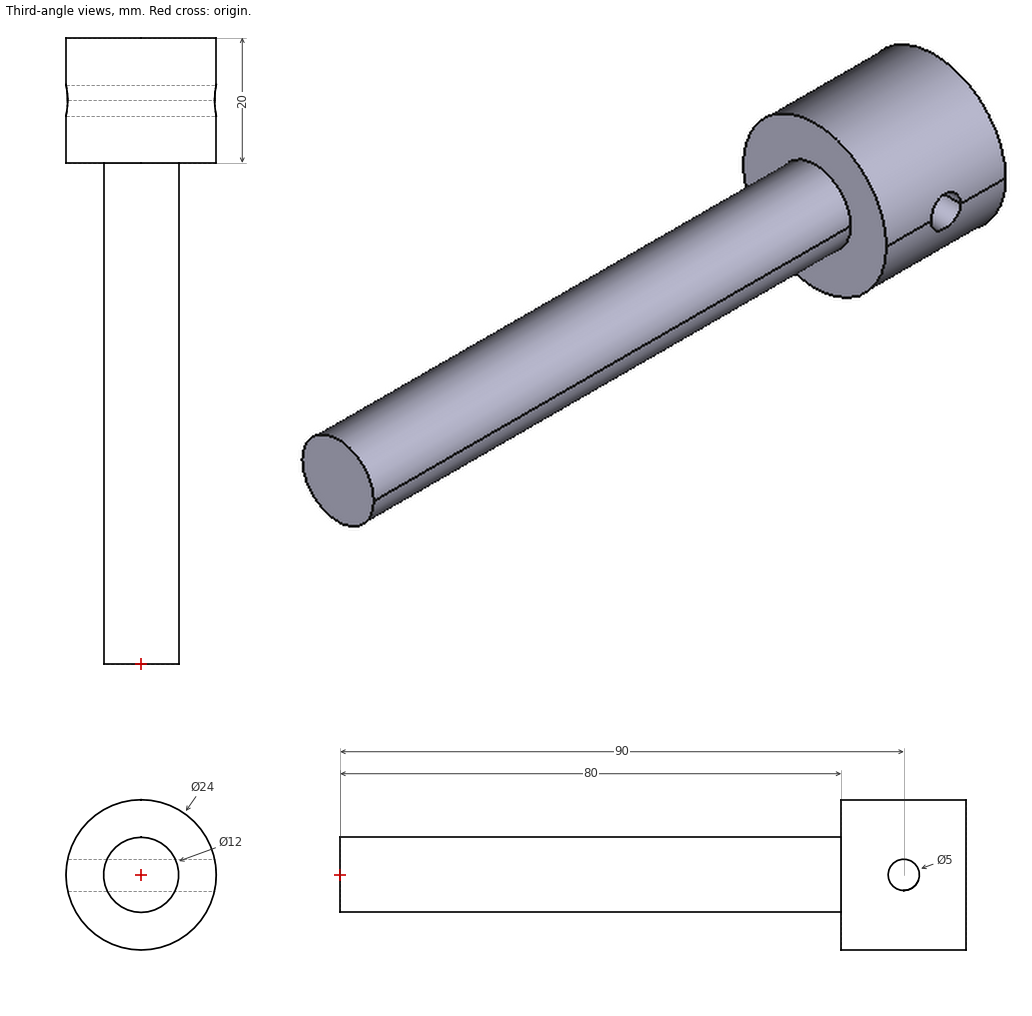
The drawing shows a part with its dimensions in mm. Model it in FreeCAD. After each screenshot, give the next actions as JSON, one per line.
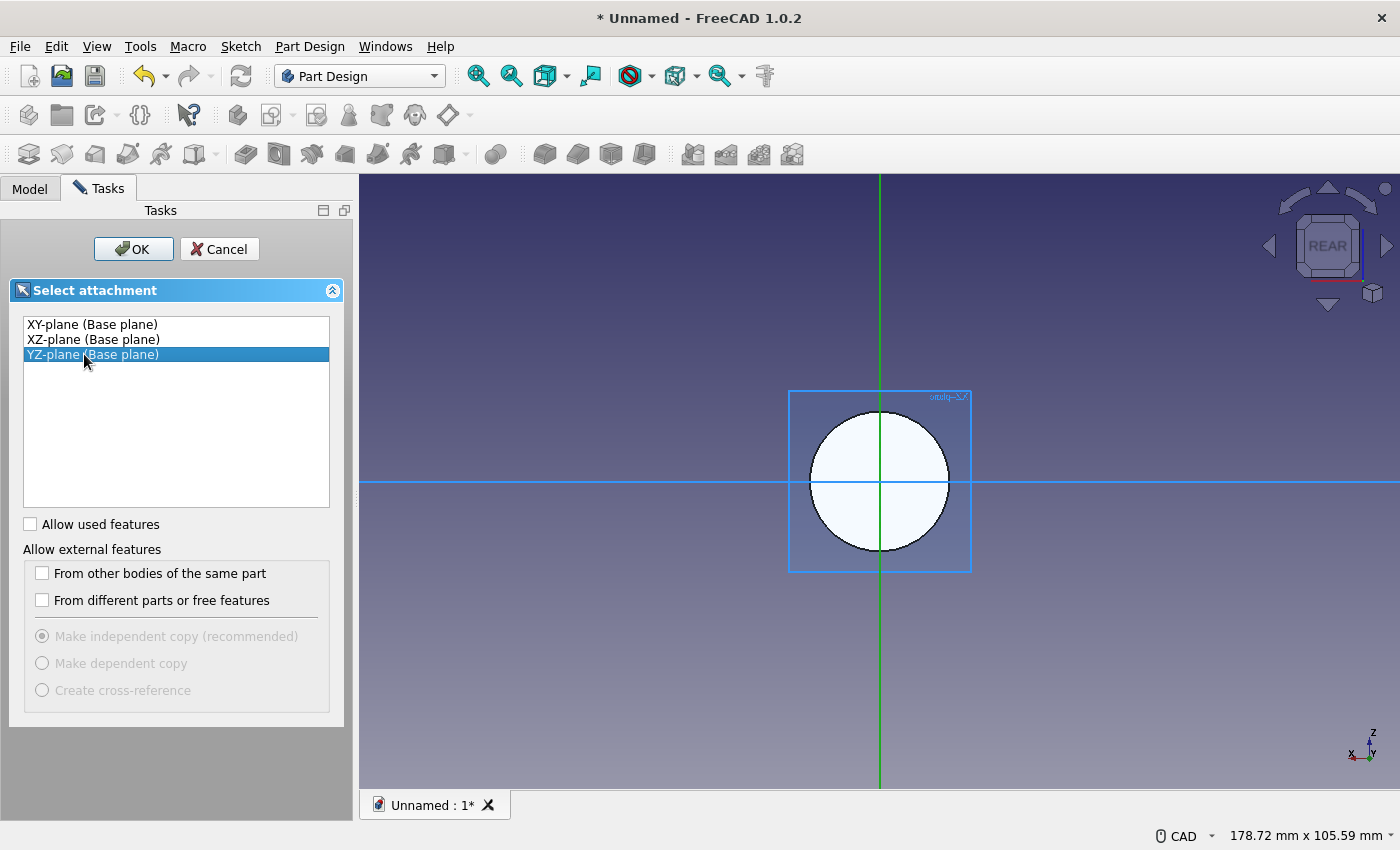
{"action": "left_click", "coordinate": [134, 249]}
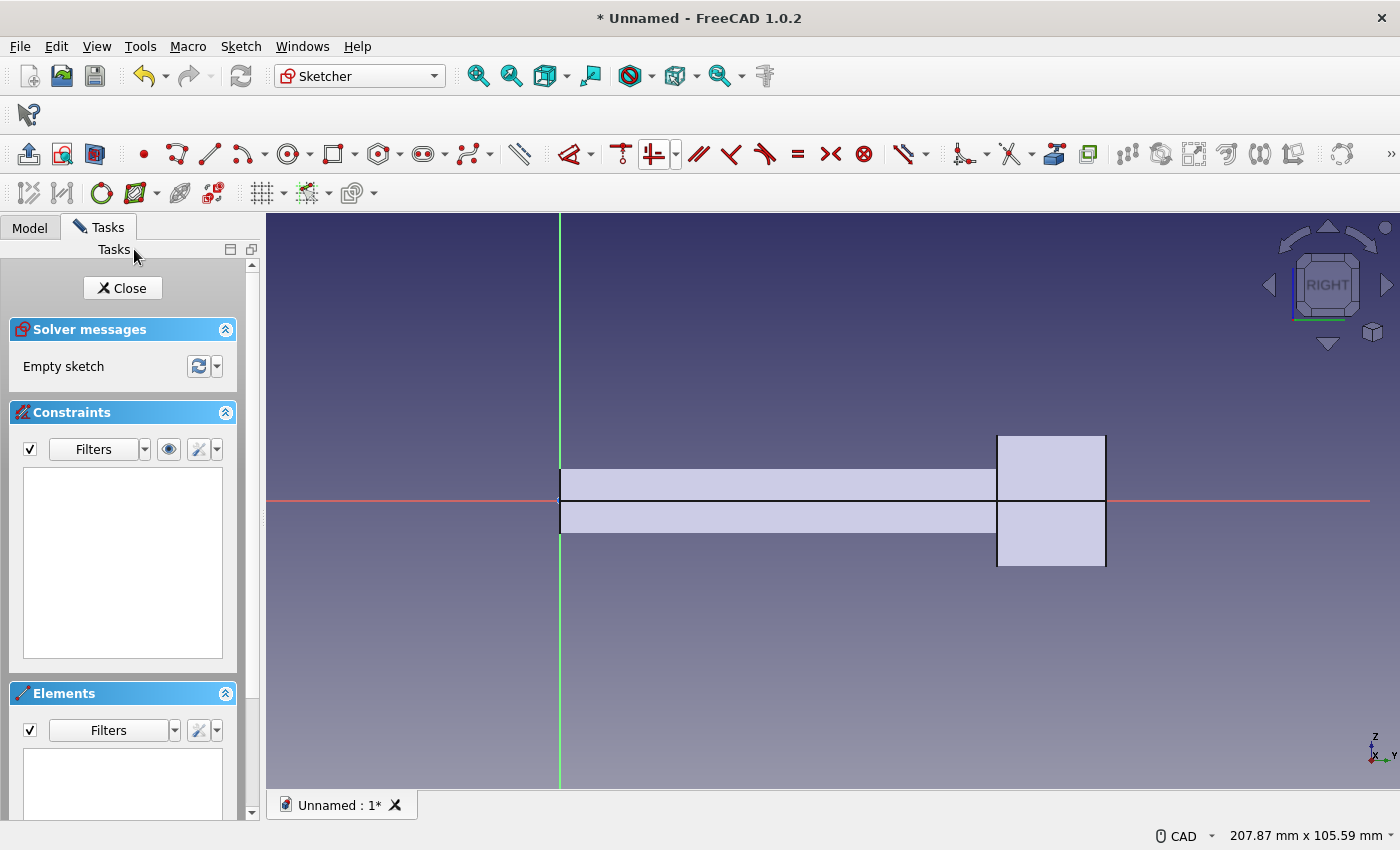
{"action": "key", "text": "q s"}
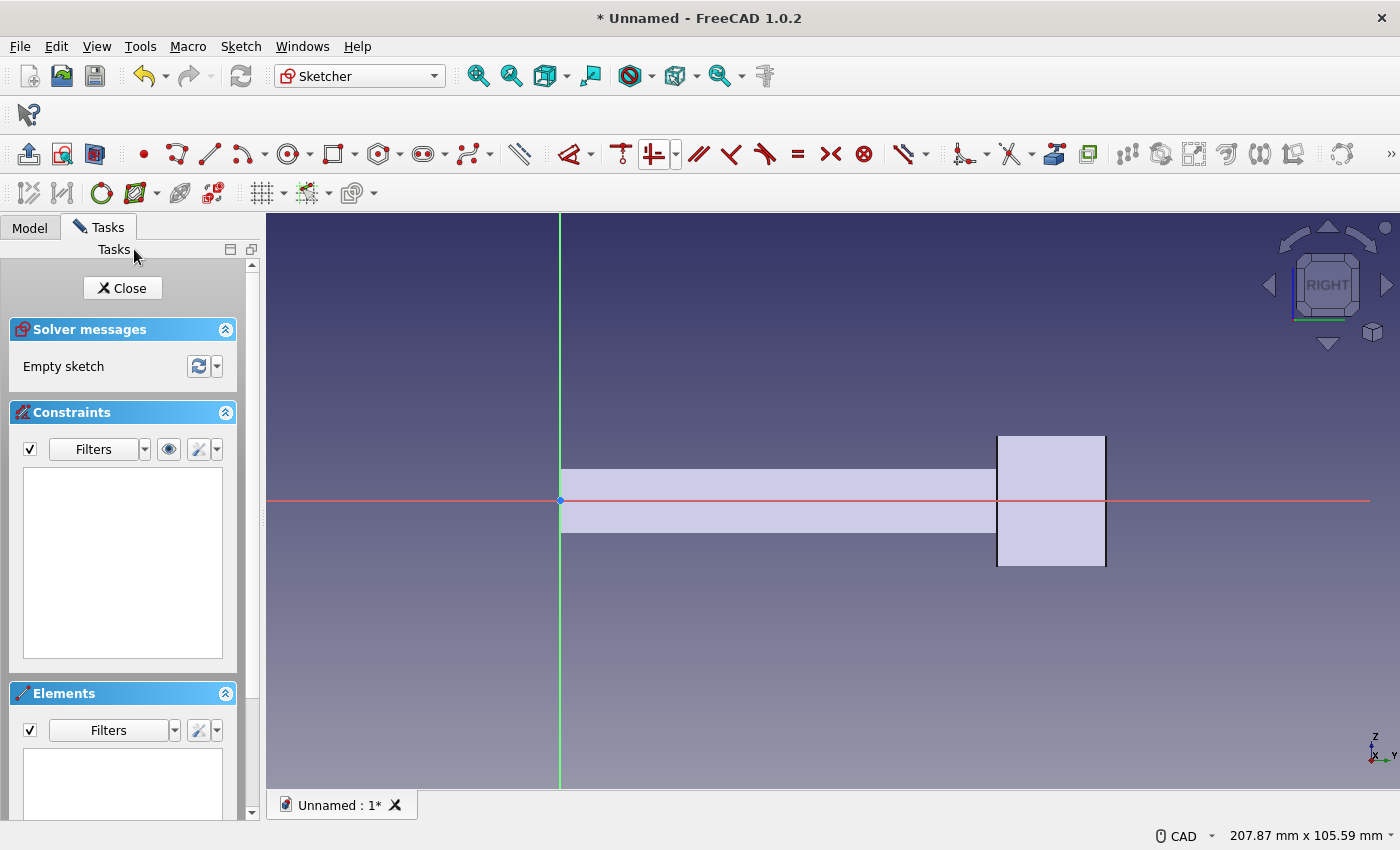
{"action": "scroll", "coordinate": [1074, 501], "scroll_direction": "up", "scroll_amount": 13}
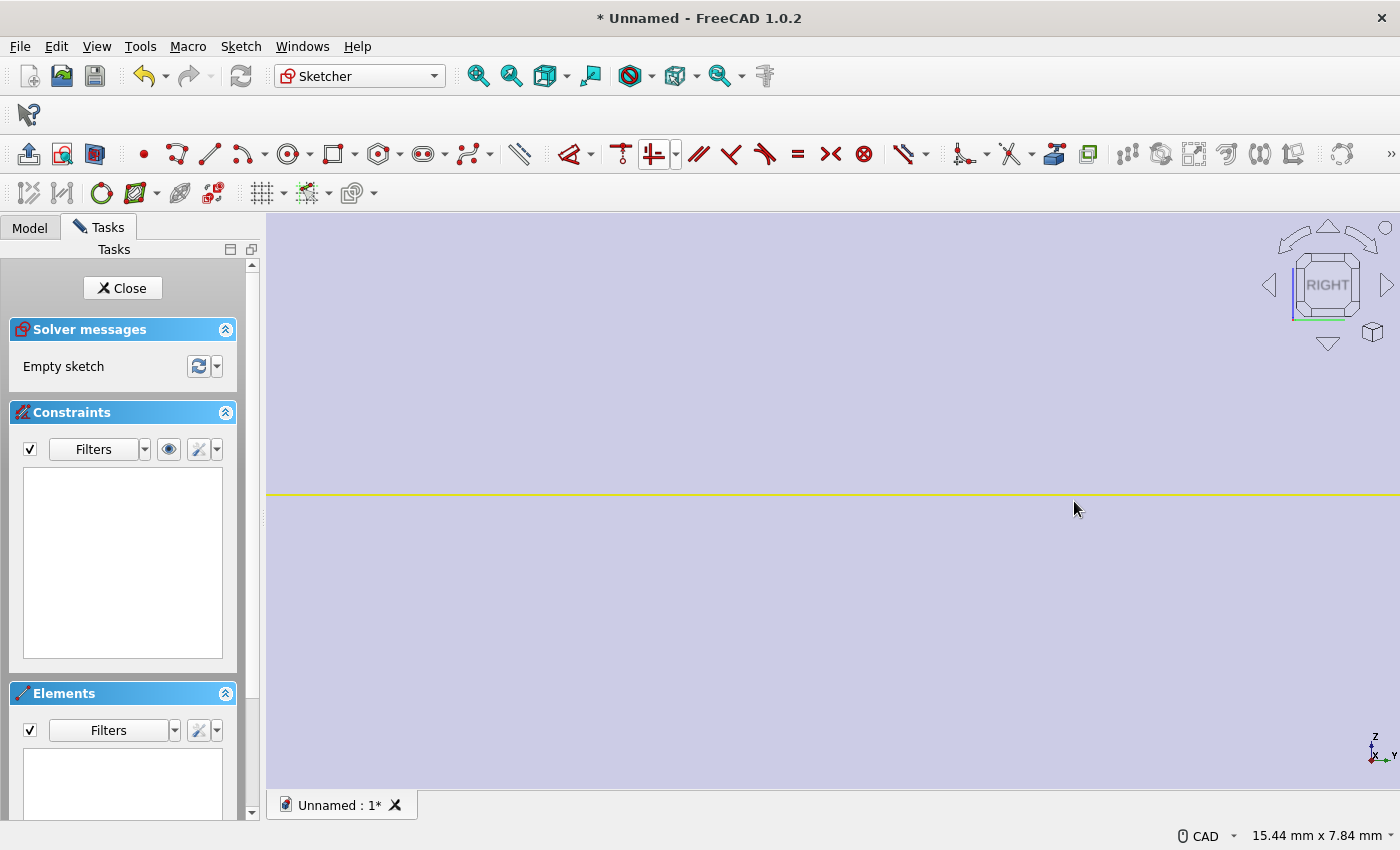
{"action": "key", "text": "g c"}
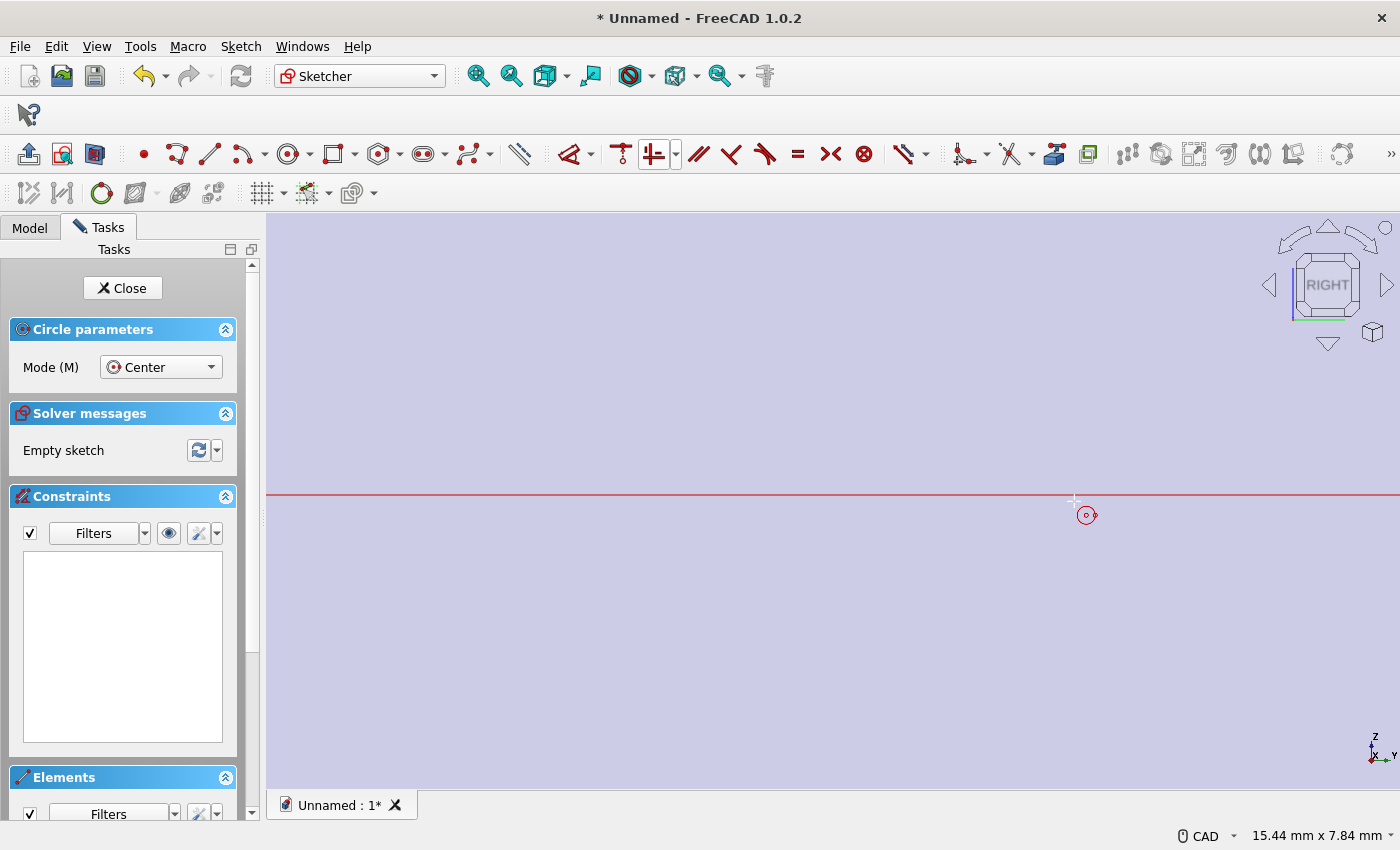
{"action": "left_click", "coordinate": [758, 495]}
{"action": "left_click", "coordinate": [888, 365]}
{"action": "key", "text": "Escape"}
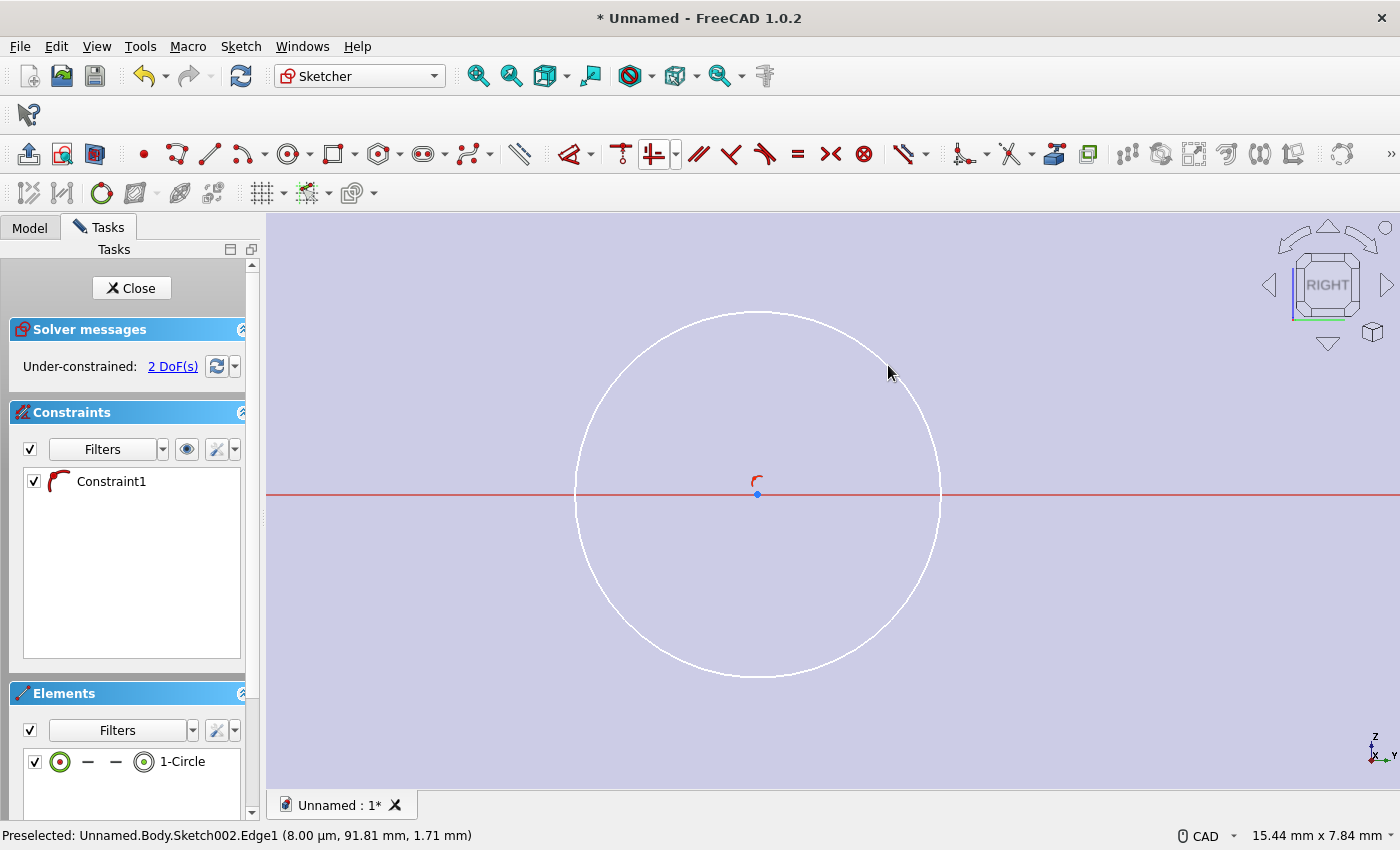
{"action": "left_click", "coordinate": [887, 365]}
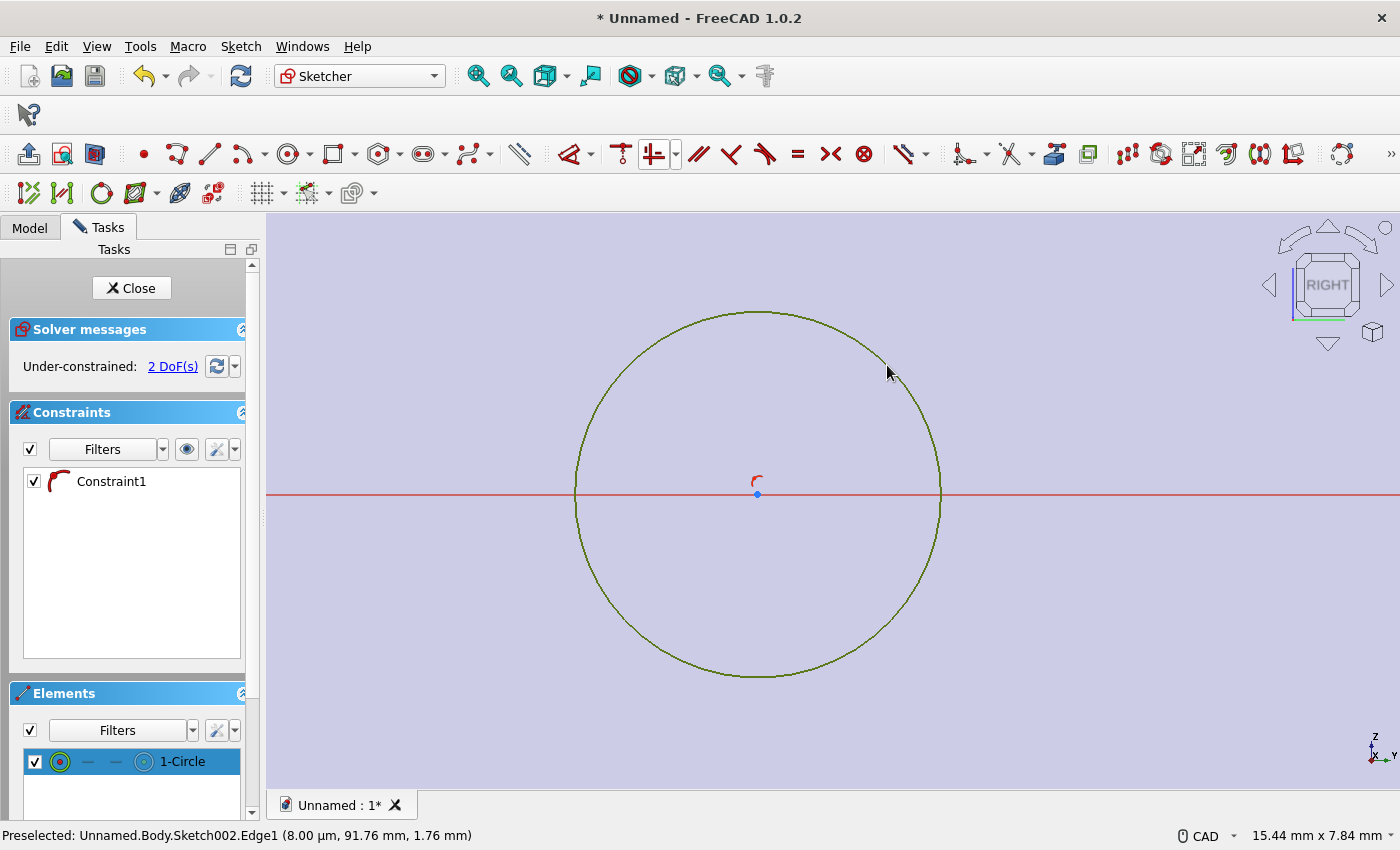
{"action": "key", "text": "k o"}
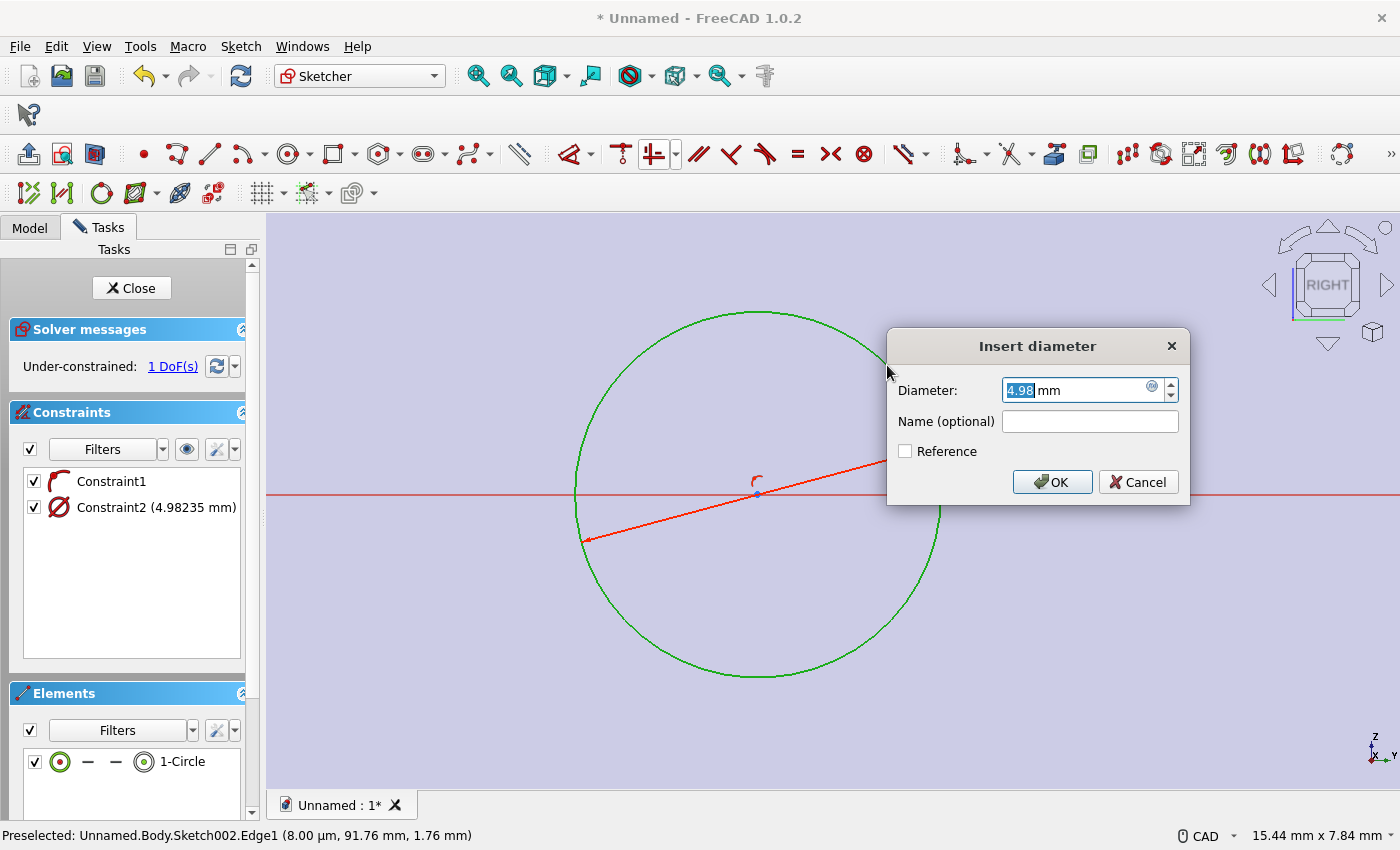
{"action": "type", "text": "5"}
{"action": "key", "text": "Return"}